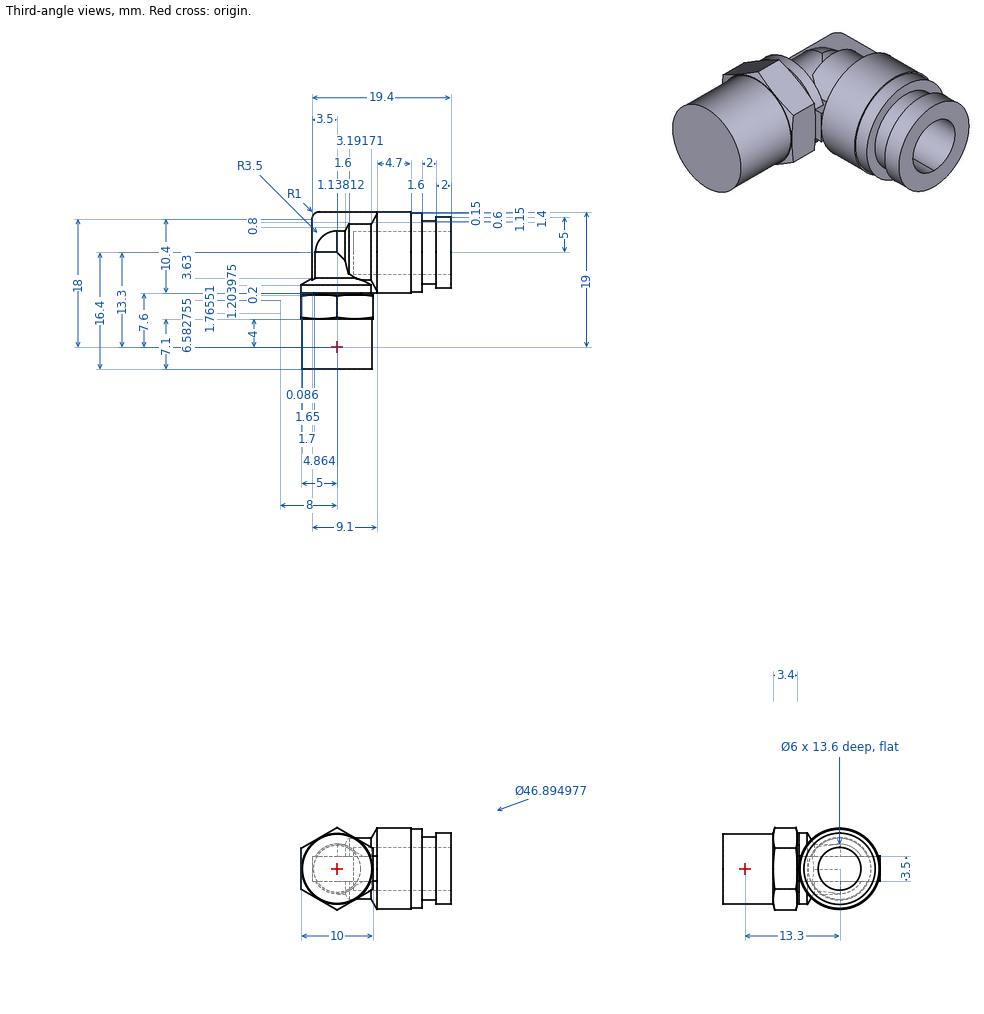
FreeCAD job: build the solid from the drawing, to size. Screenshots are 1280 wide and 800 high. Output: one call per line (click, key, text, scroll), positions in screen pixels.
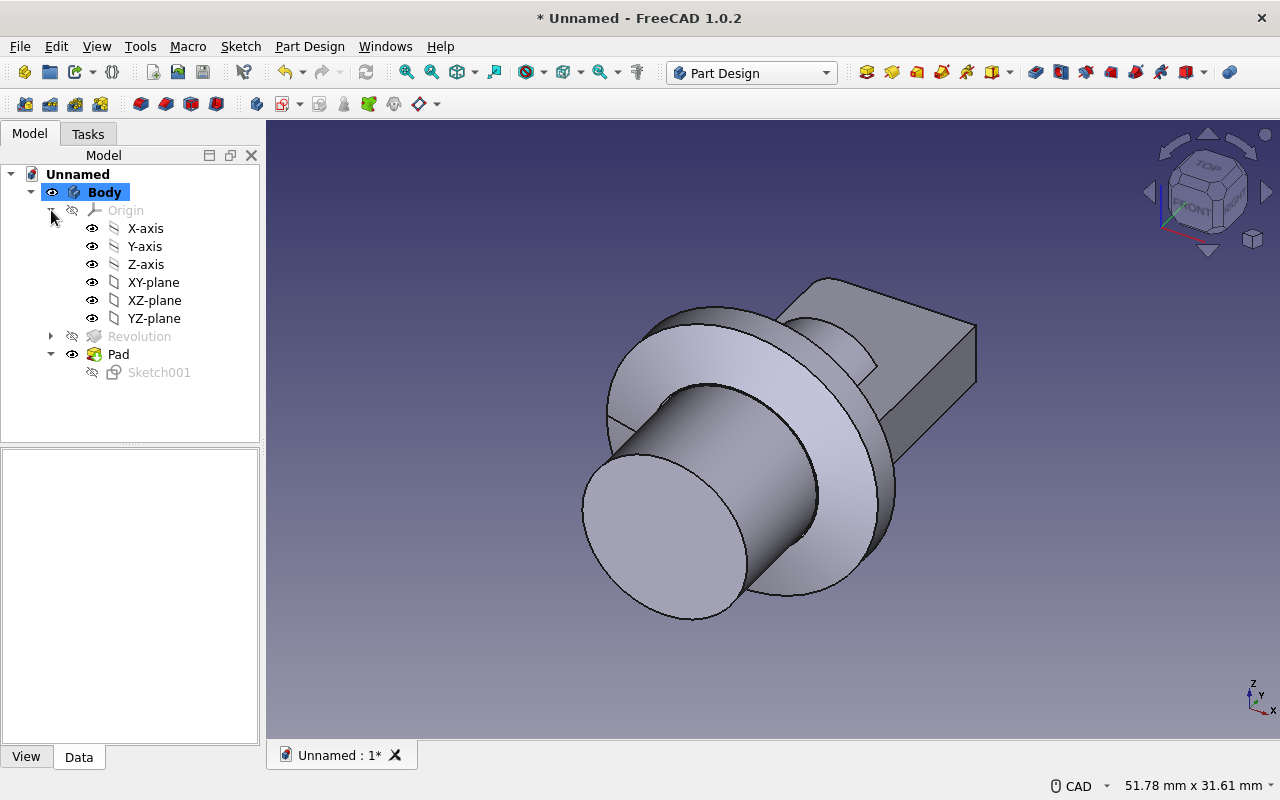
click(137, 300)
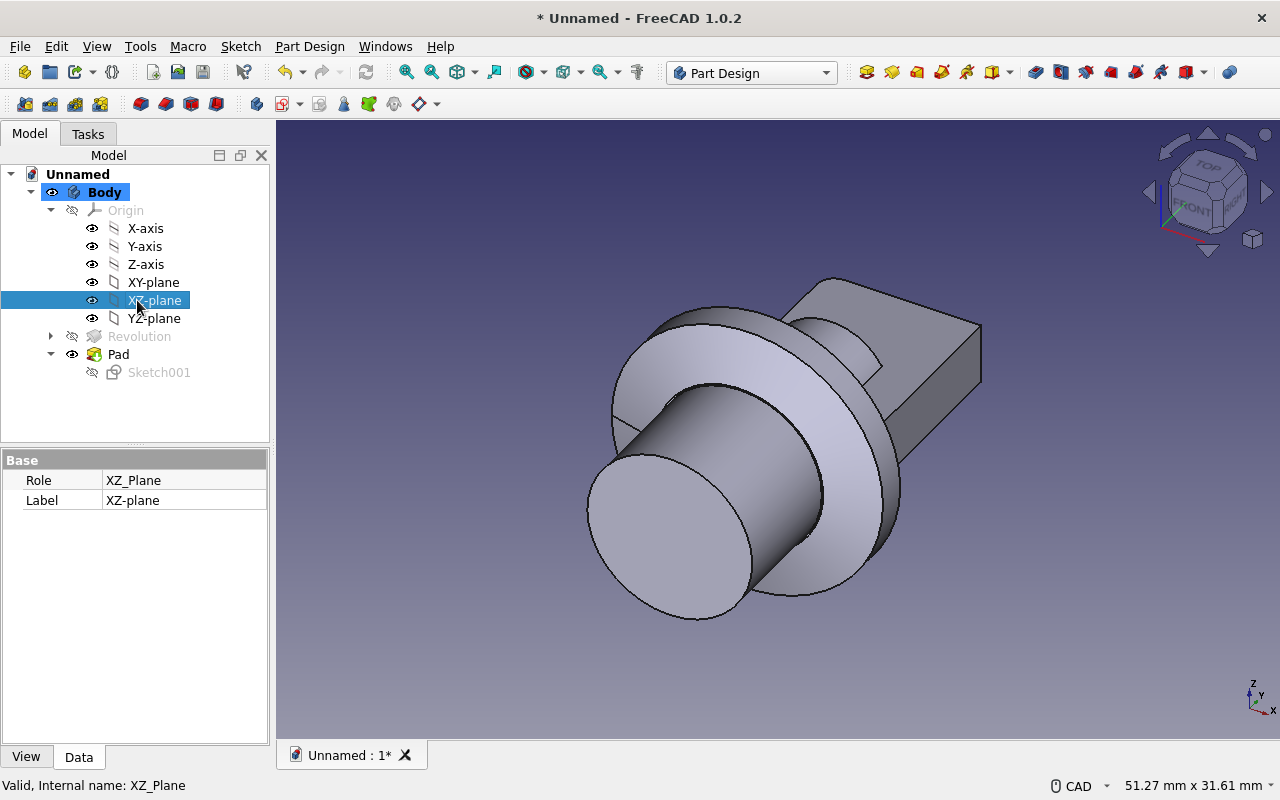
click(418, 104)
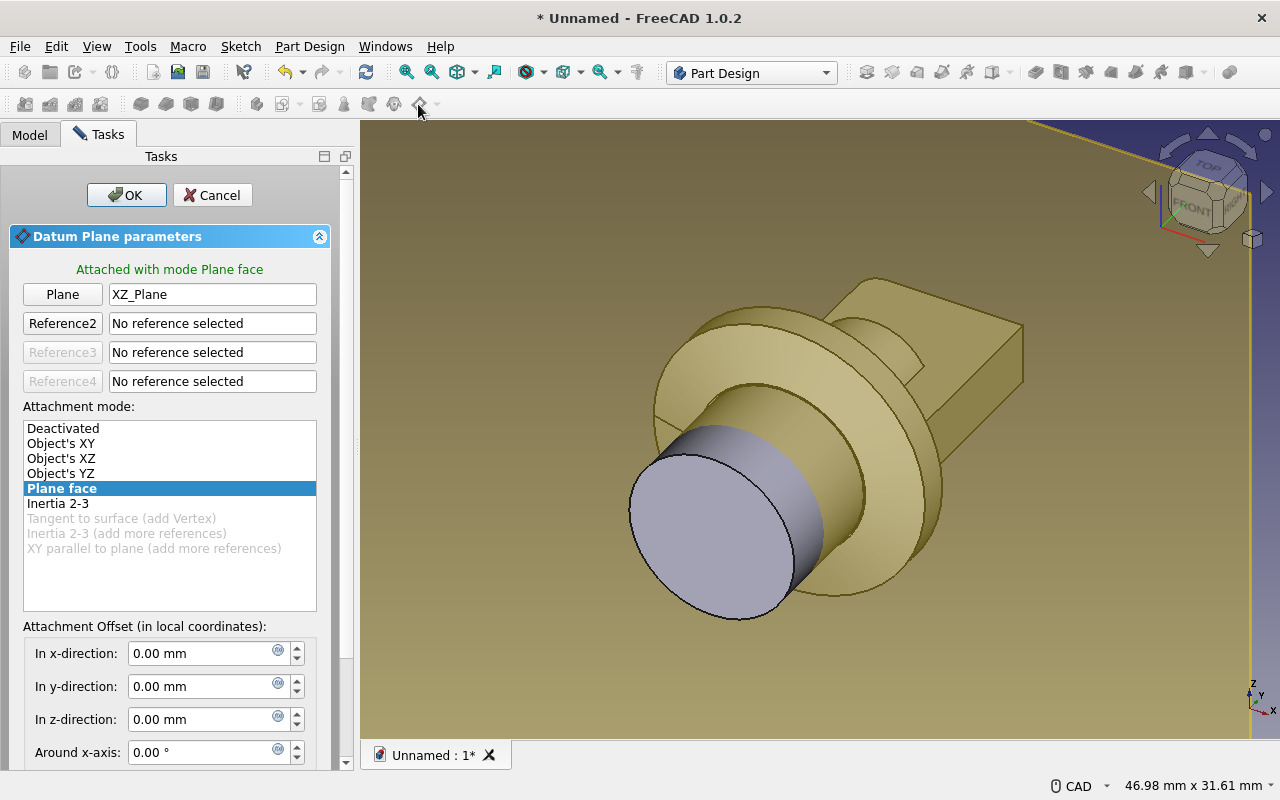
triple_click(210, 720)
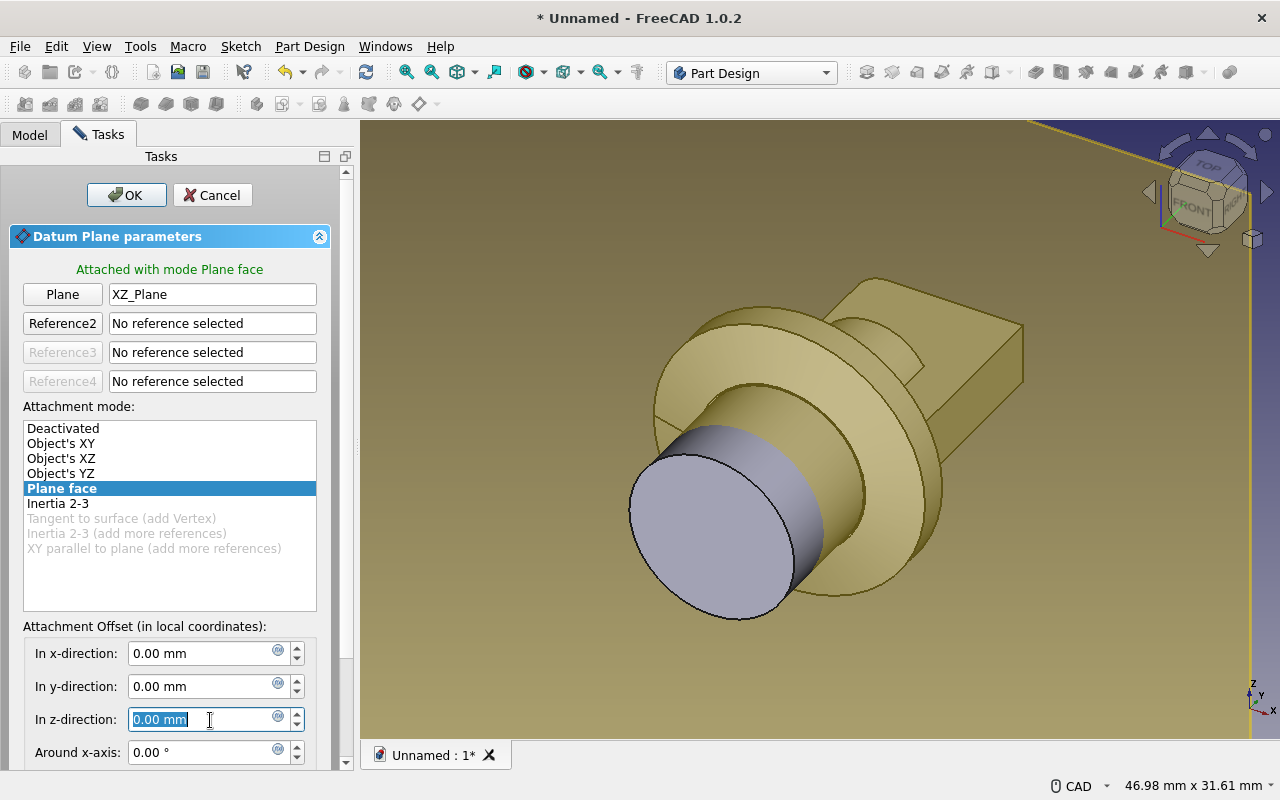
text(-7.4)
key(Tab)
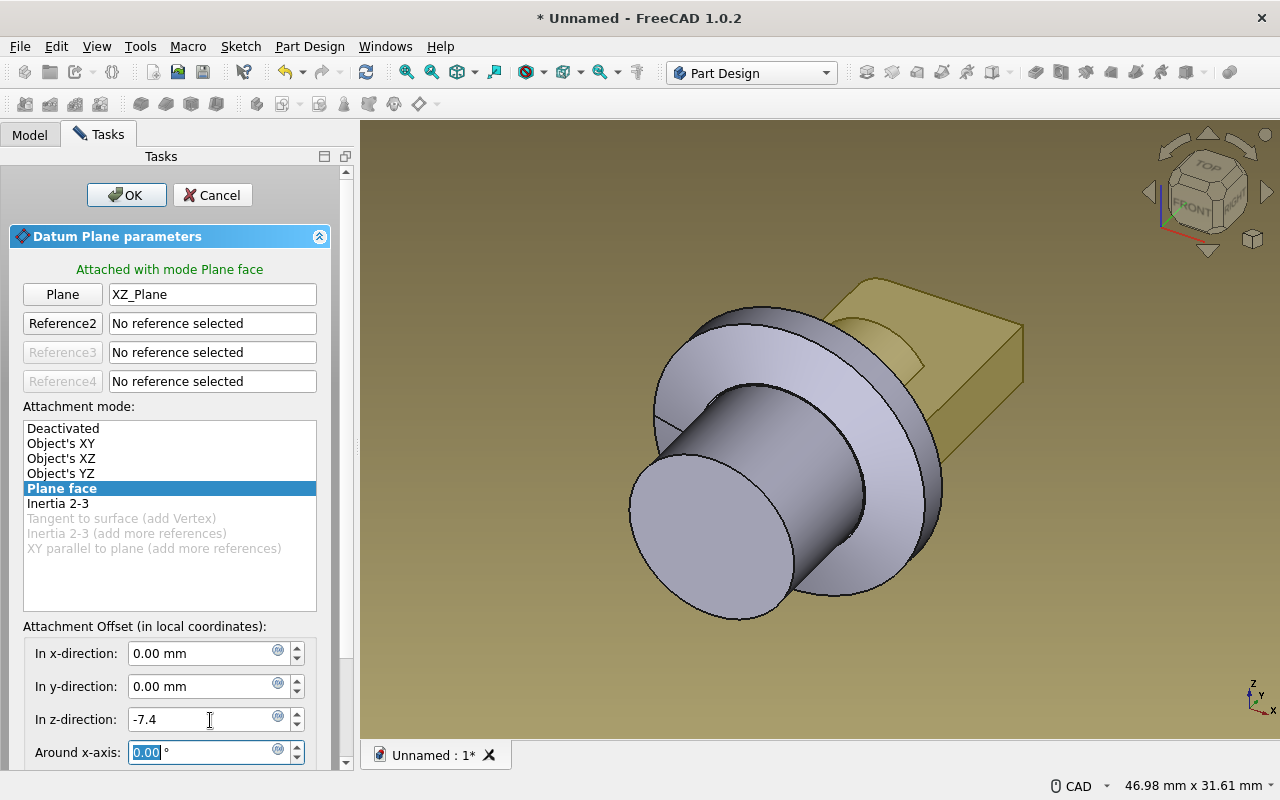
click(127, 195)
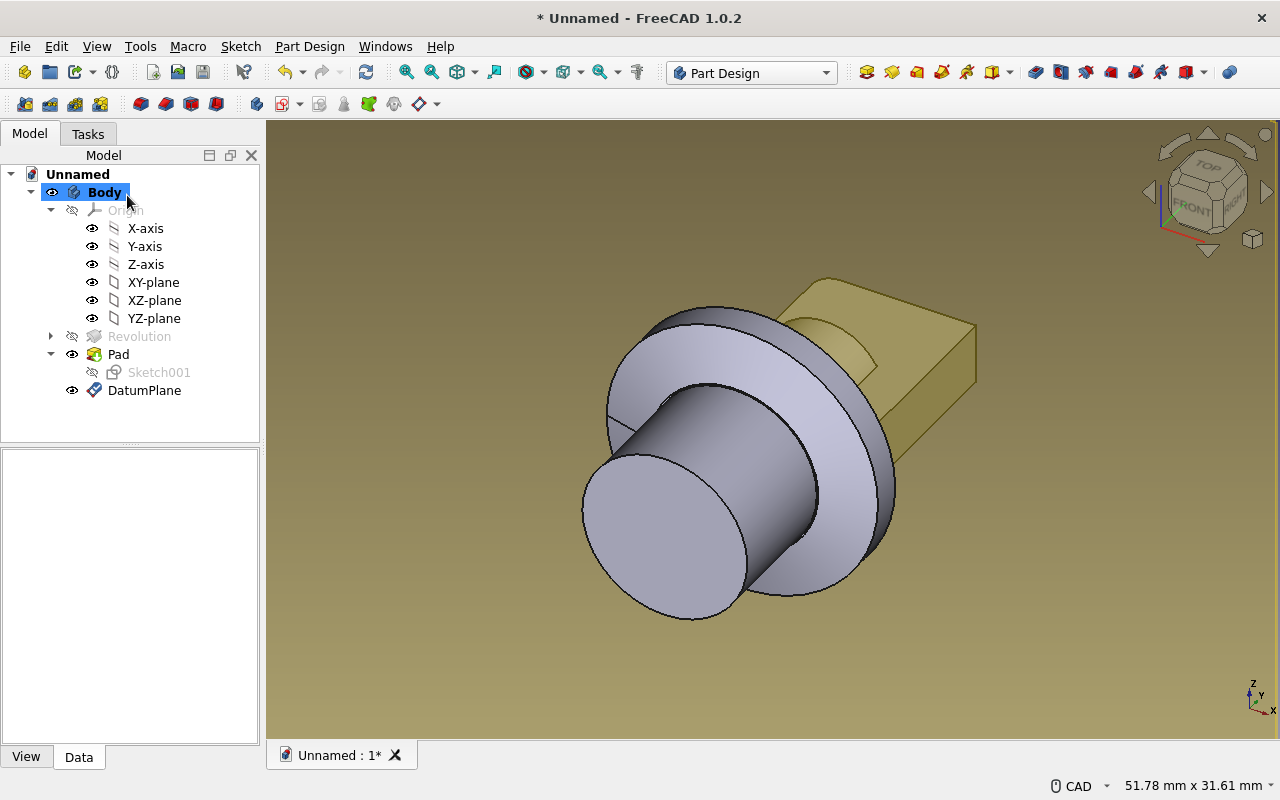
click(117, 390)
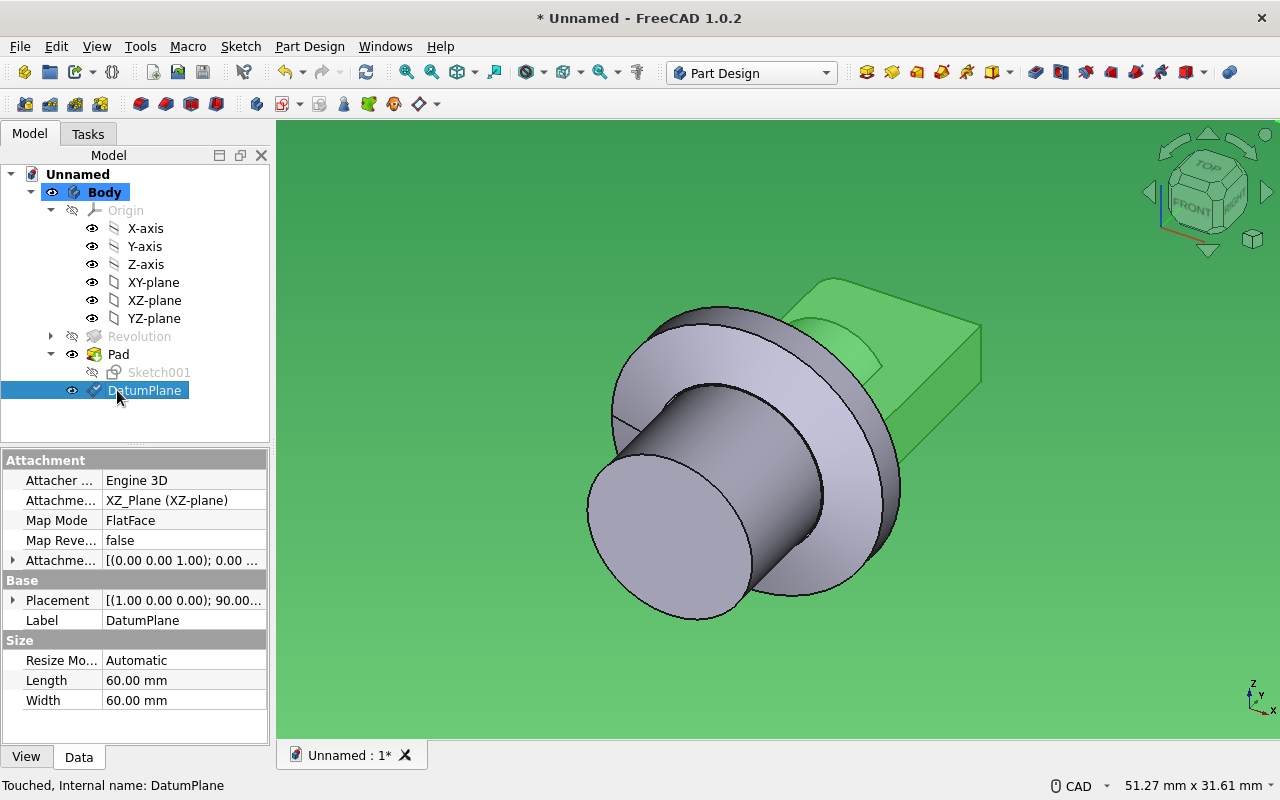
click(282, 104)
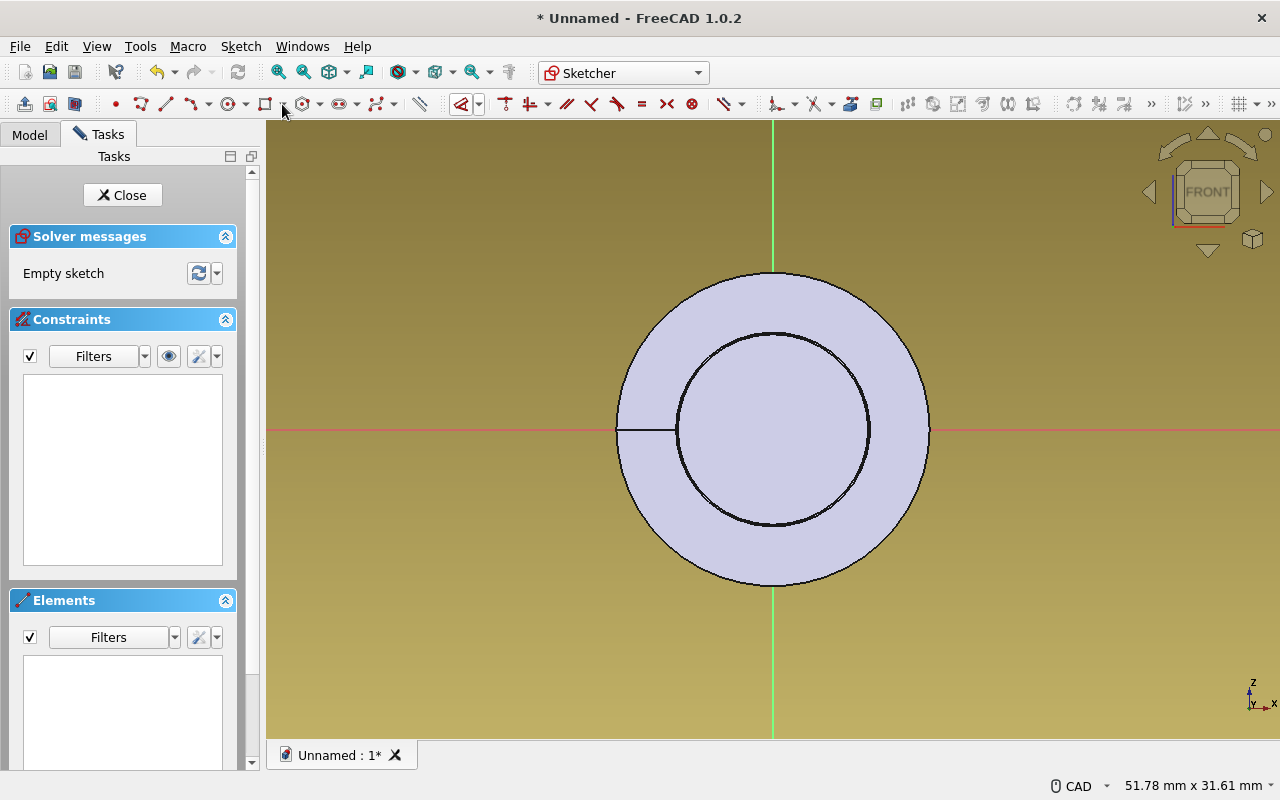
click(75, 104)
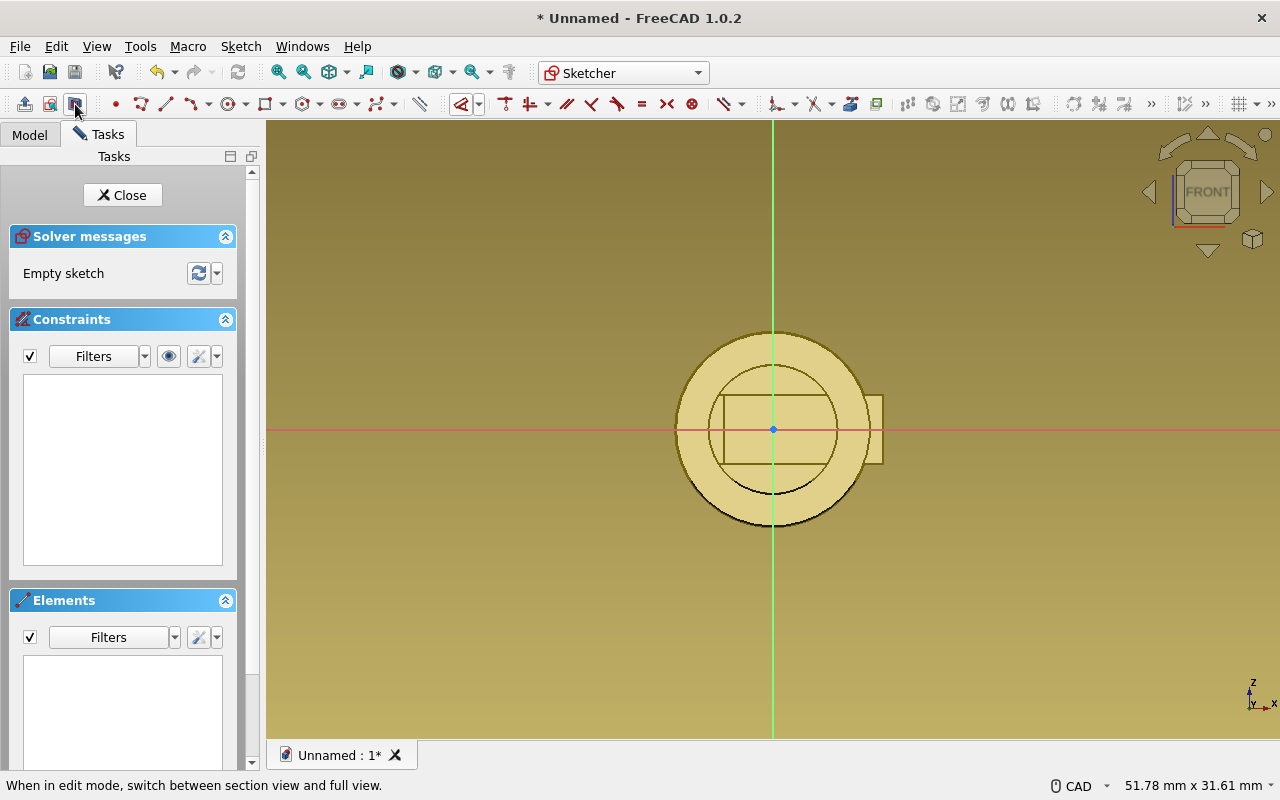
scroll(649, 429, down, 4)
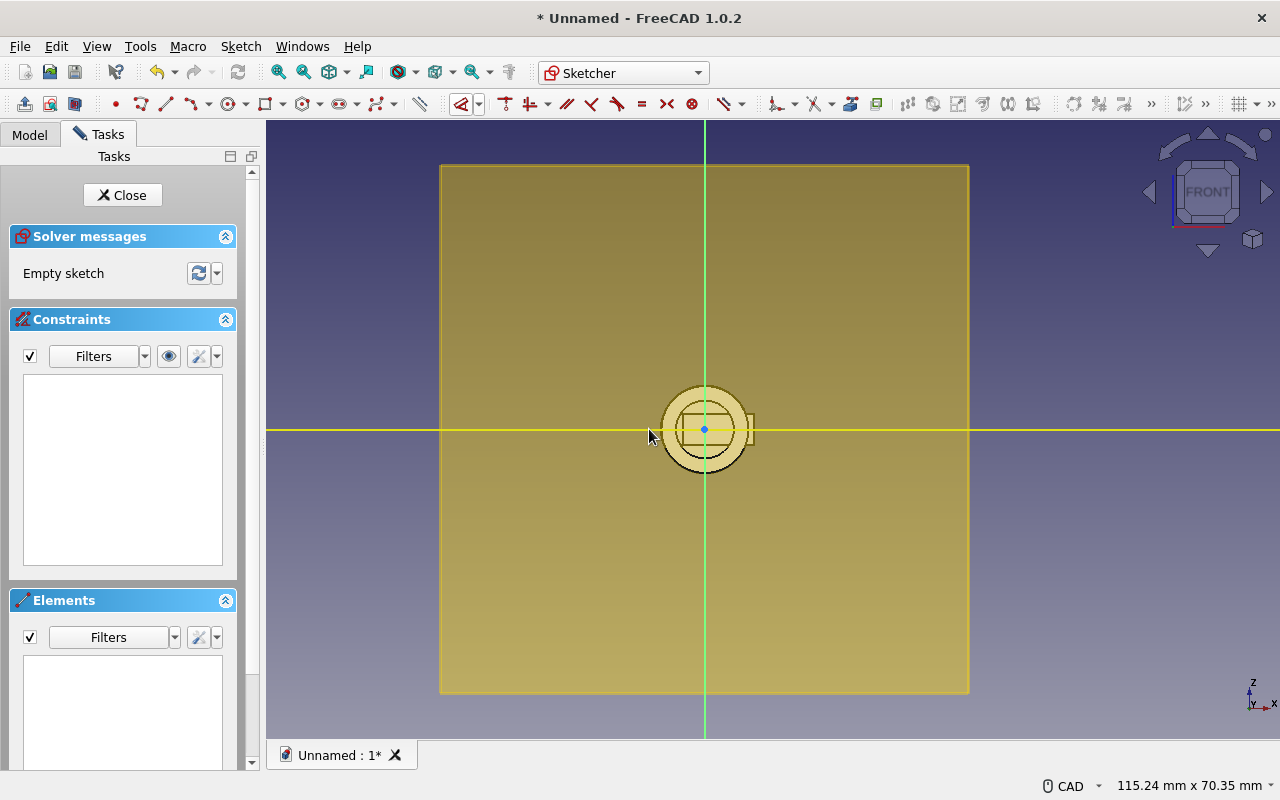
key(g)
key(p)
key(6)